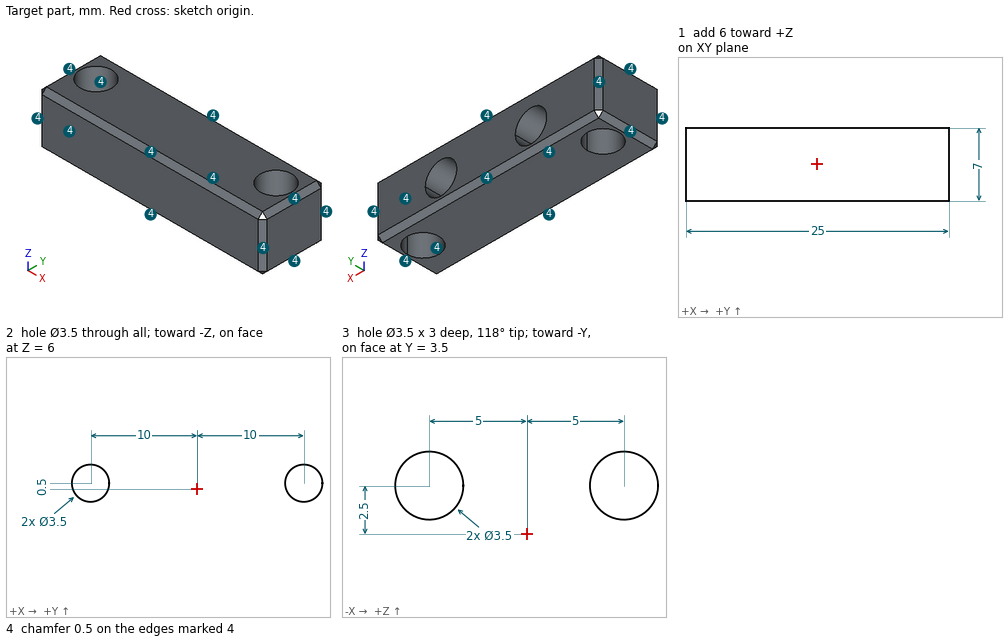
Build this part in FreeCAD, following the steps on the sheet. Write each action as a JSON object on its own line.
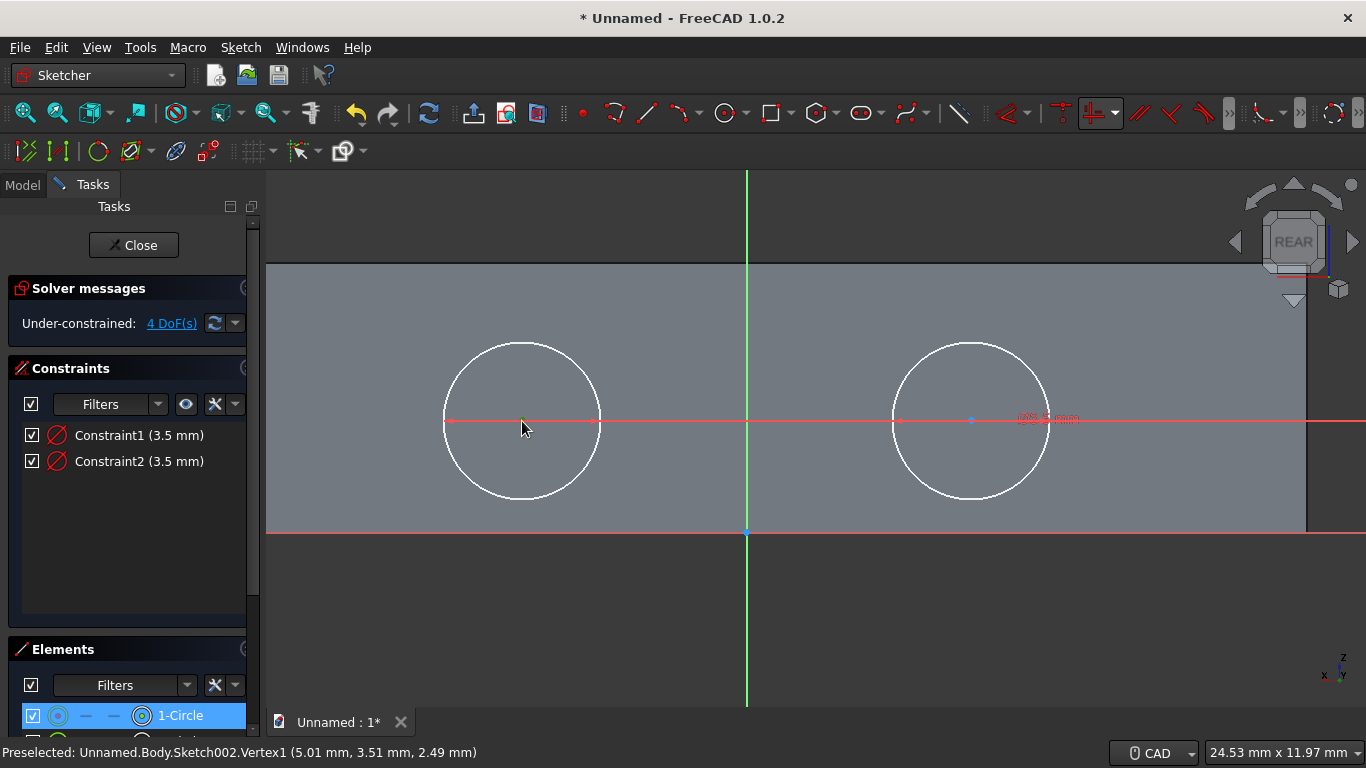
{"action": "left_click", "coordinate": [971, 421]}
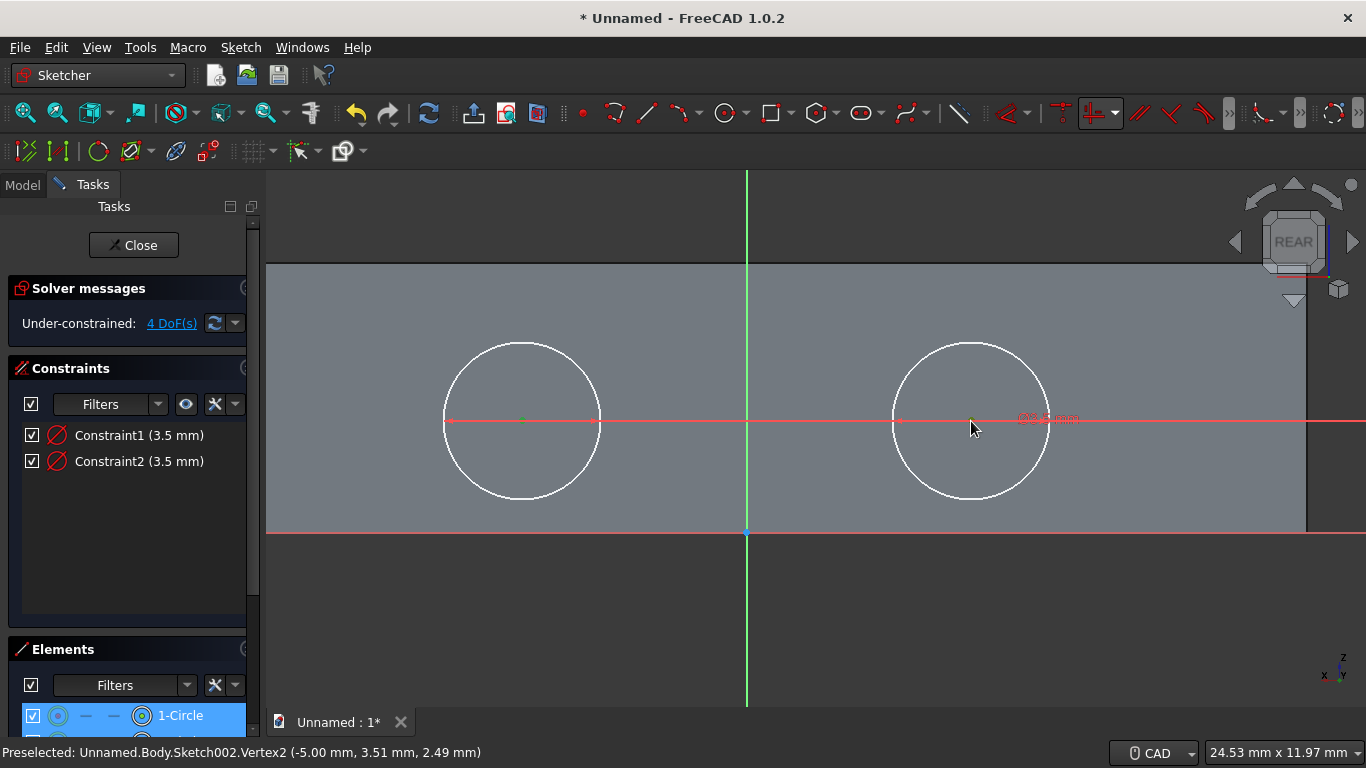
{"action": "left_click", "coordinate": [1118, 114]}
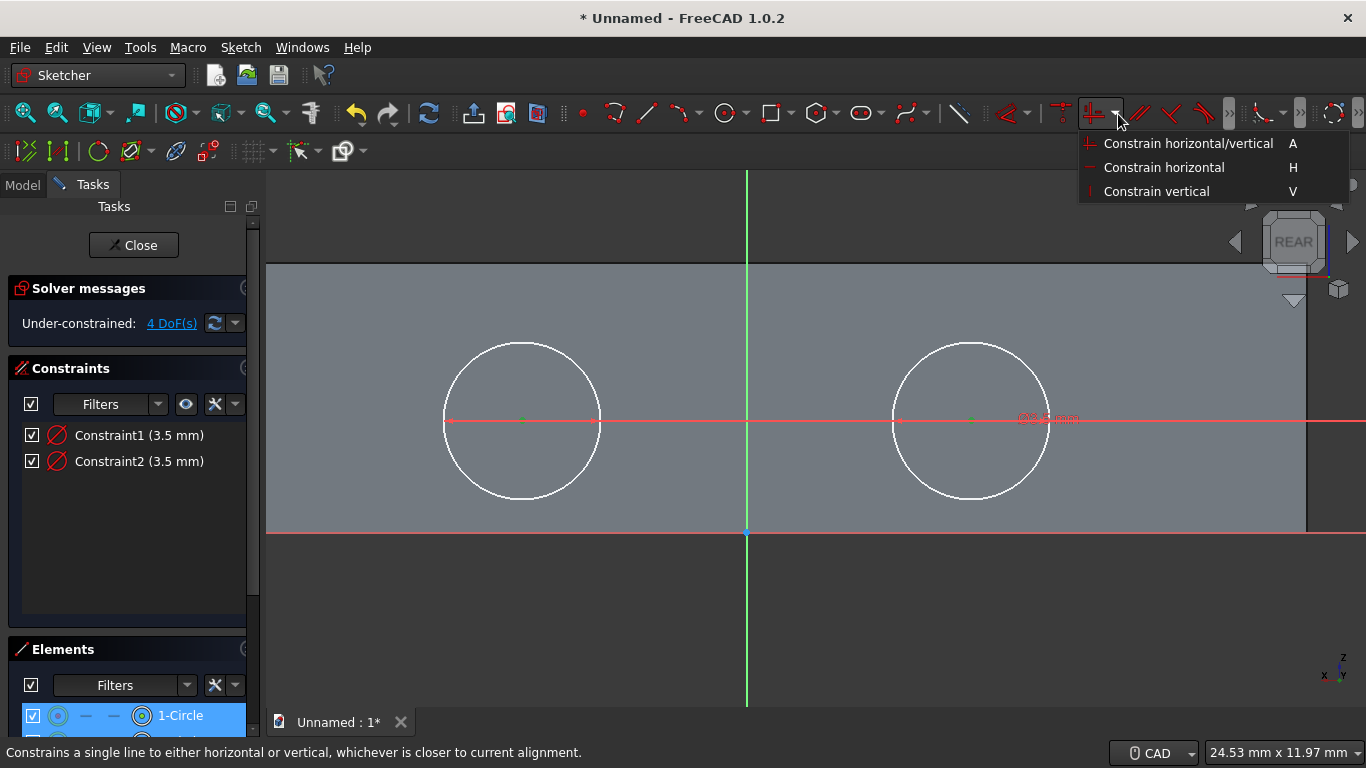
{"action": "left_click", "coordinate": [1214, 167]}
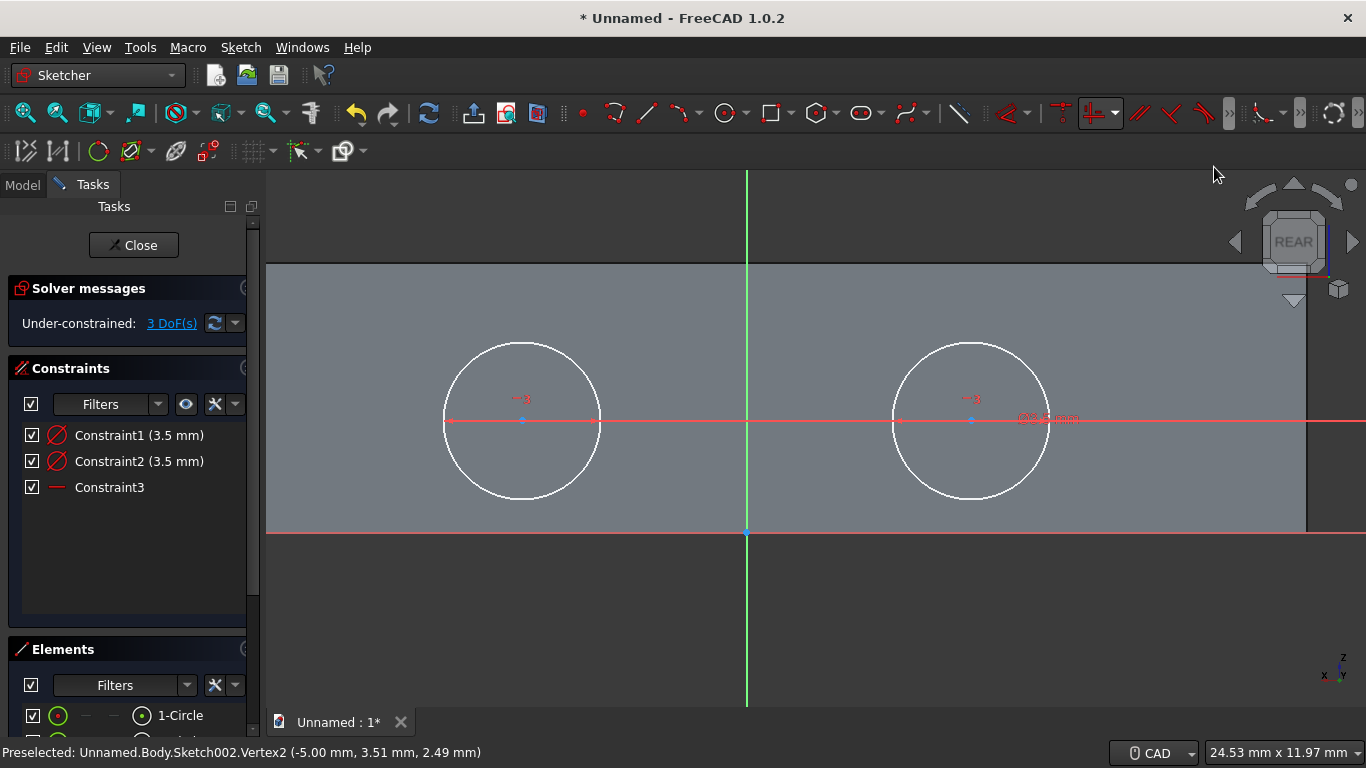
{"action": "left_click", "coordinate": [1006, 114]}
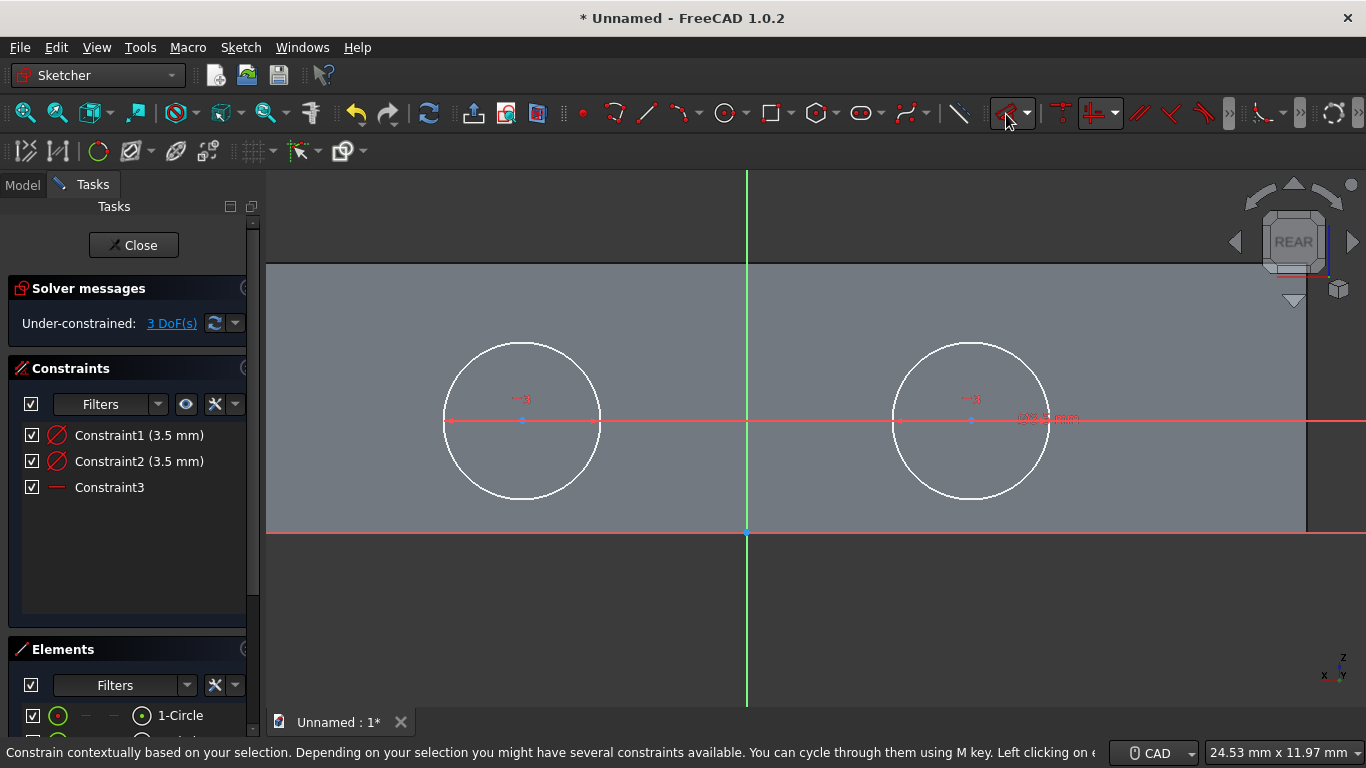
{"action": "left_click", "coordinate": [522, 421]}
{"action": "left_click", "coordinate": [634, 567]}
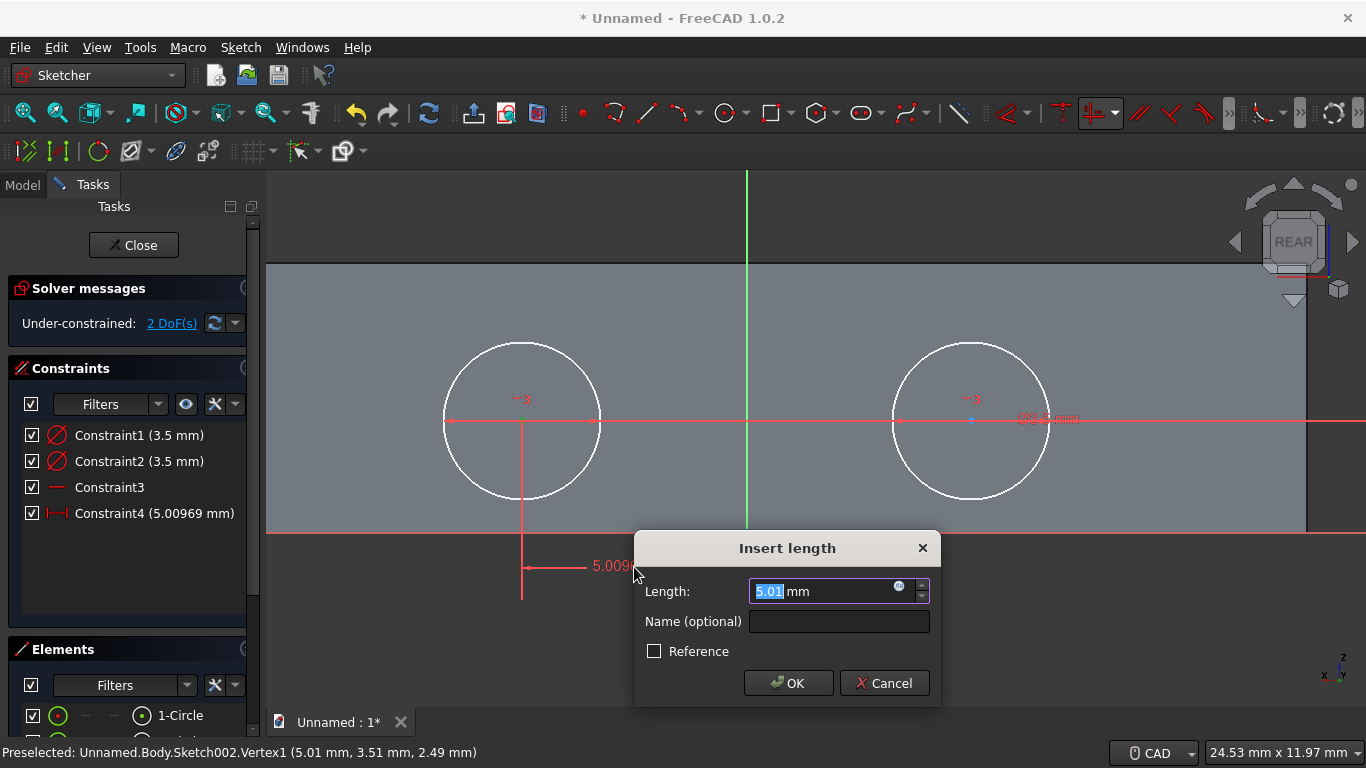
{"action": "type", "text": "5"}
{"action": "key", "text": "Return"}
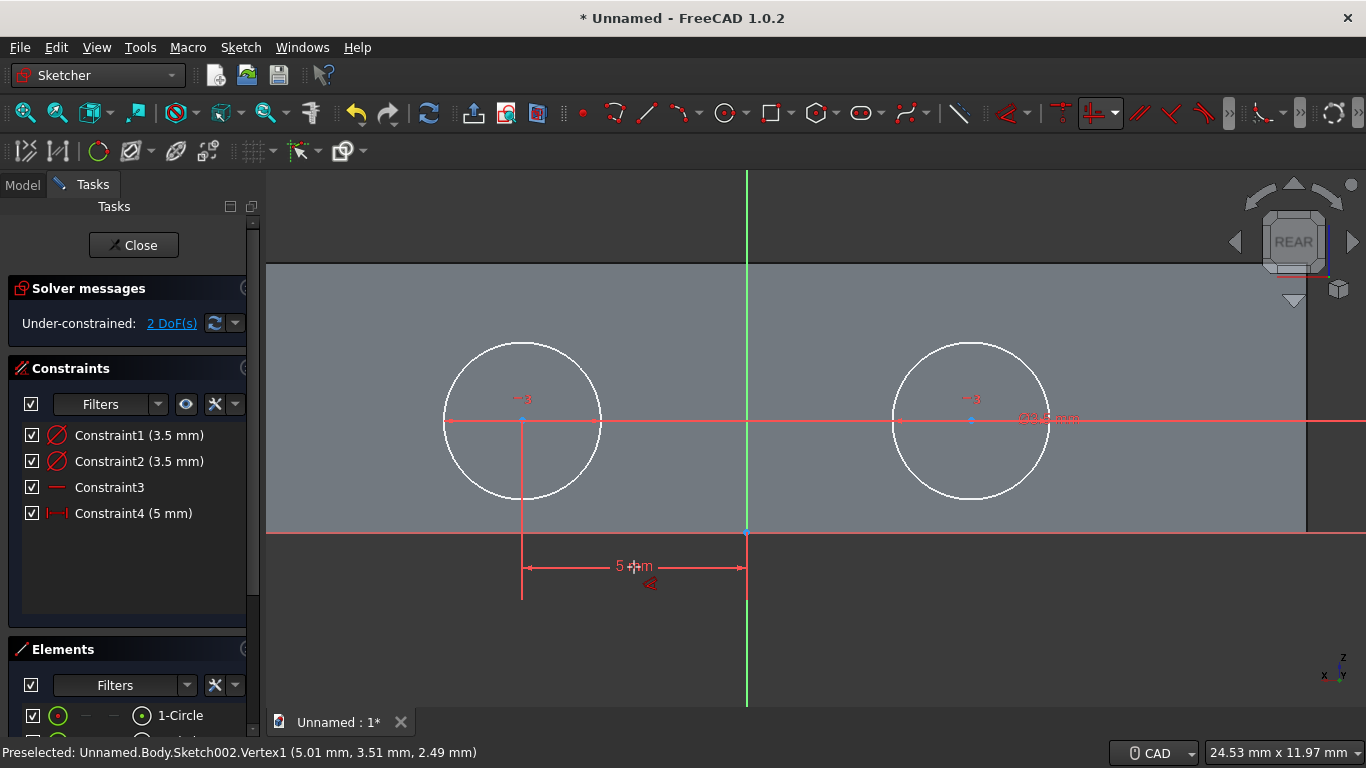
{"action": "left_click", "coordinate": [971, 421]}
{"action": "left_click", "coordinate": [859, 567]}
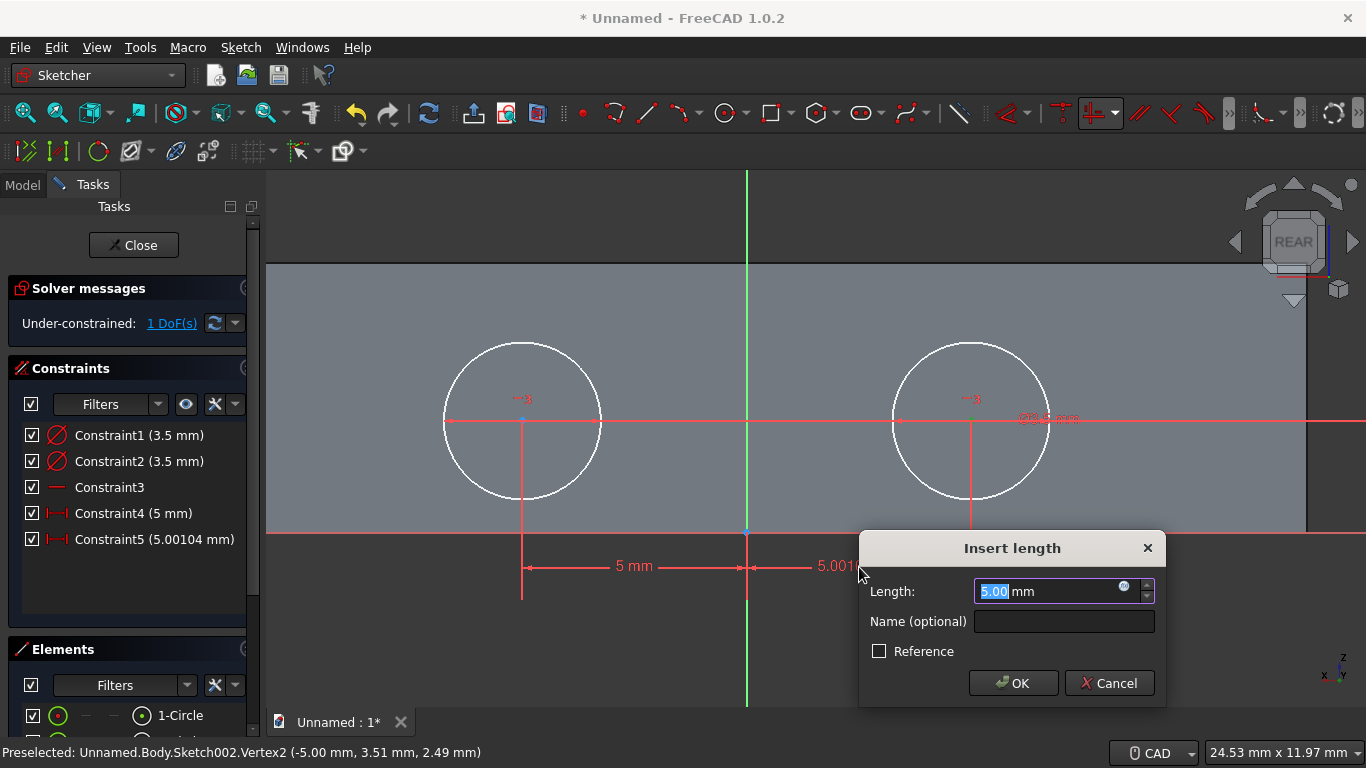
{"action": "type", "text": "5"}
{"action": "key", "text": "Return"}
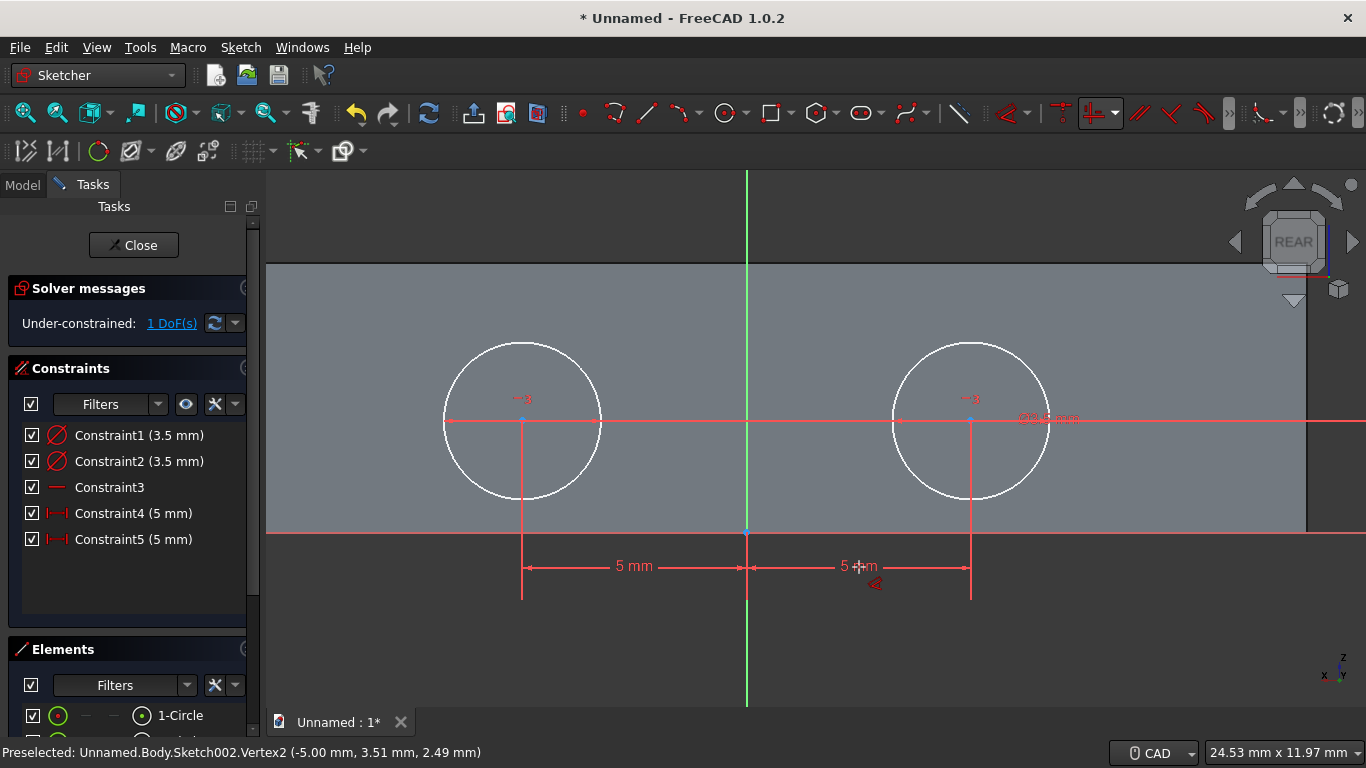
{"action": "left_click", "coordinate": [522, 421]}
{"action": "left_click", "coordinate": [488, 477]}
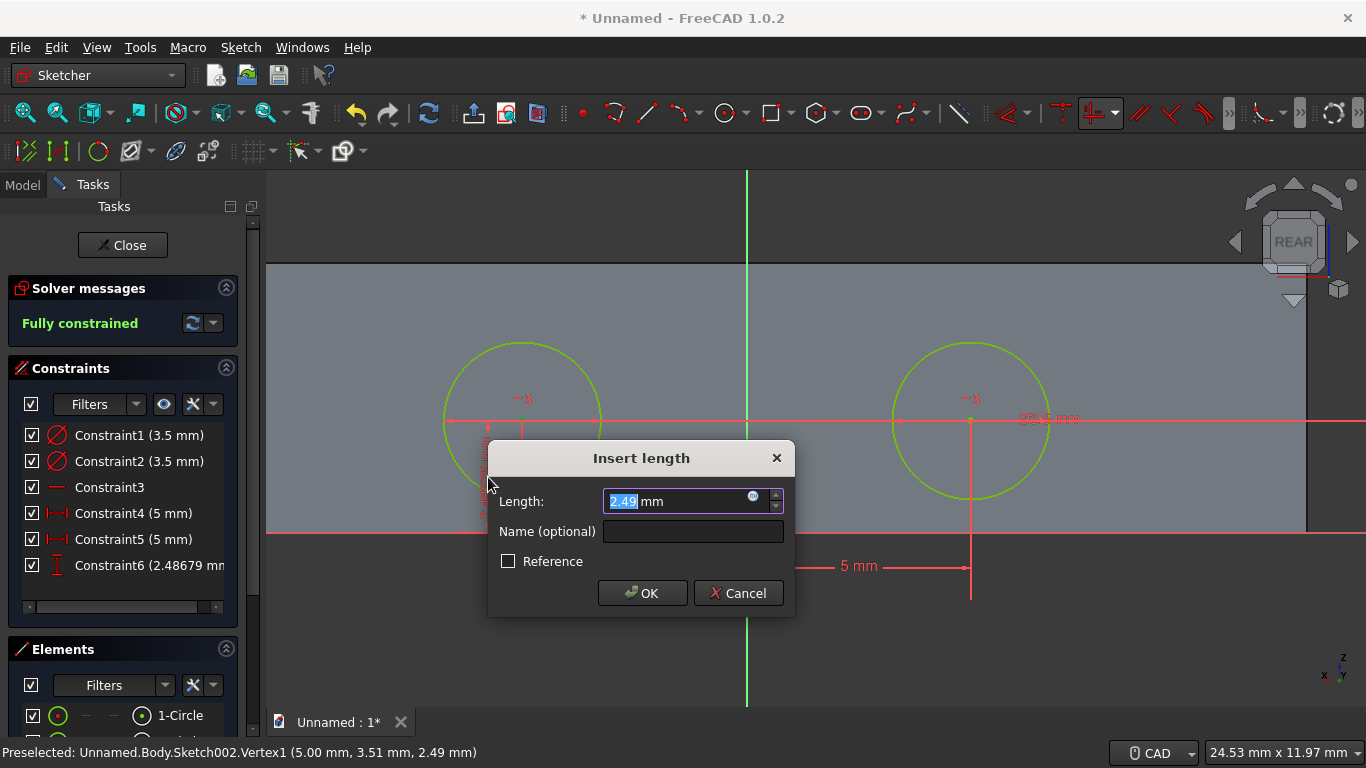
{"action": "type", "text": "2.5"}
{"action": "key", "text": "Return"}
{"action": "key", "text": "Escape"}